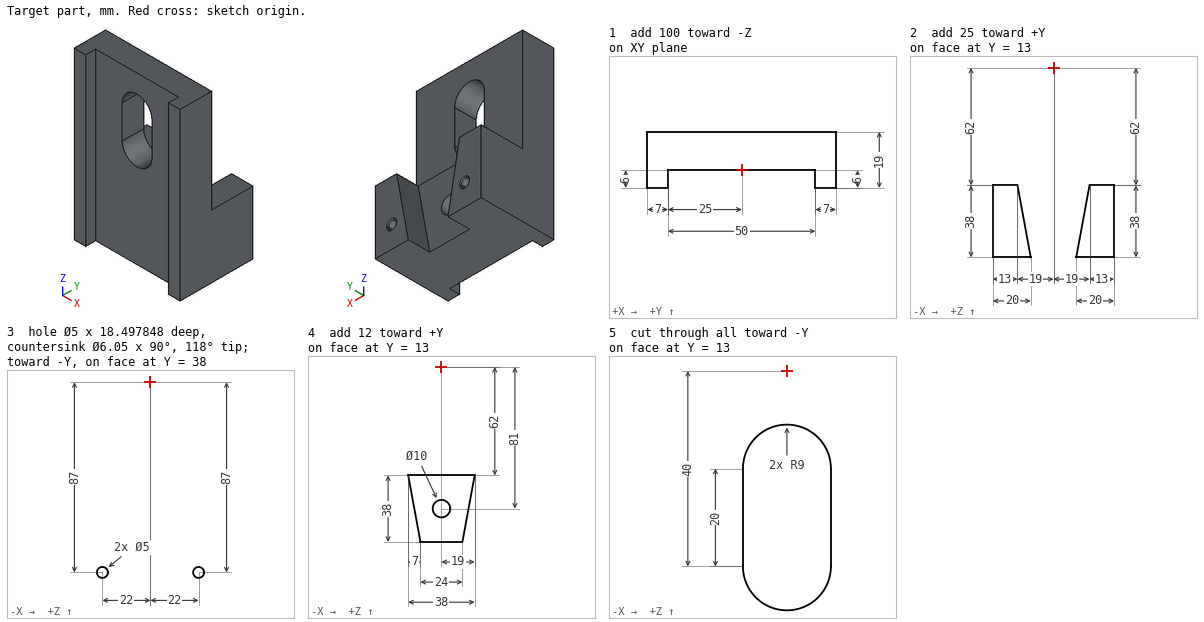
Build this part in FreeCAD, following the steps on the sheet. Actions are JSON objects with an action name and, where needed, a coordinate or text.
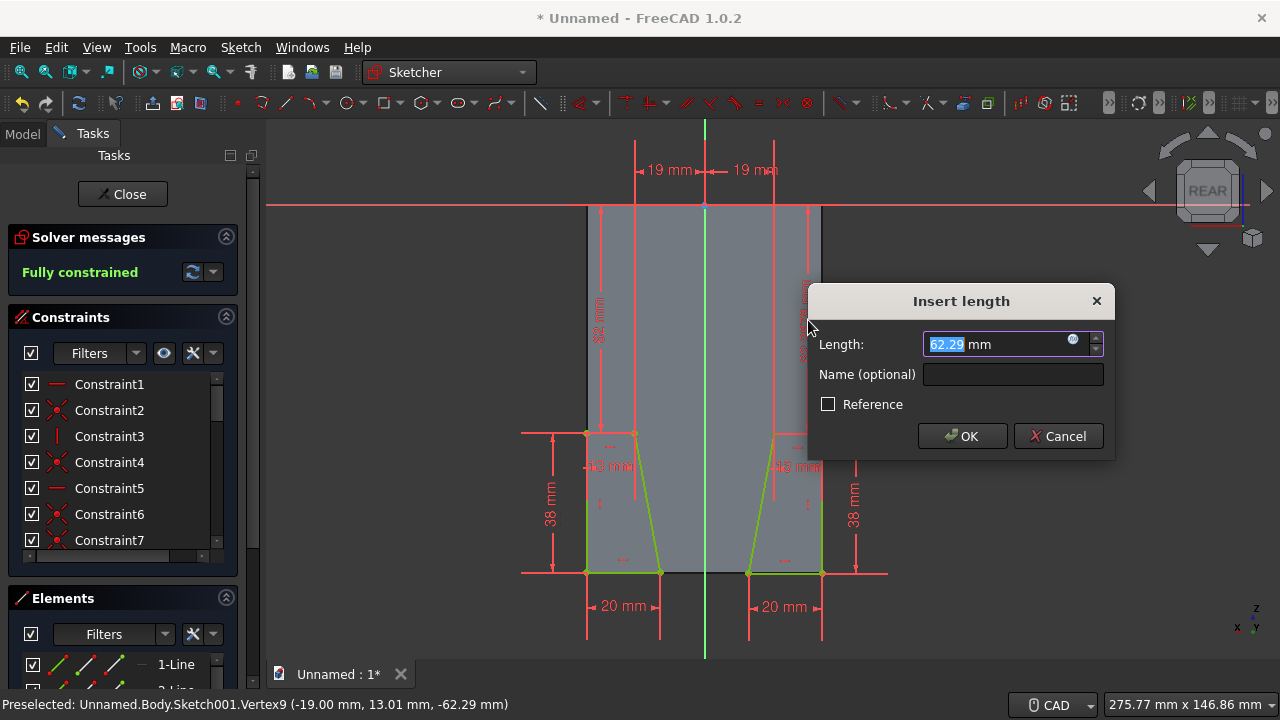
{"action": "type", "text": "62"}
{"action": "key", "text": "Return"}
{"action": "key", "text": "Escape"}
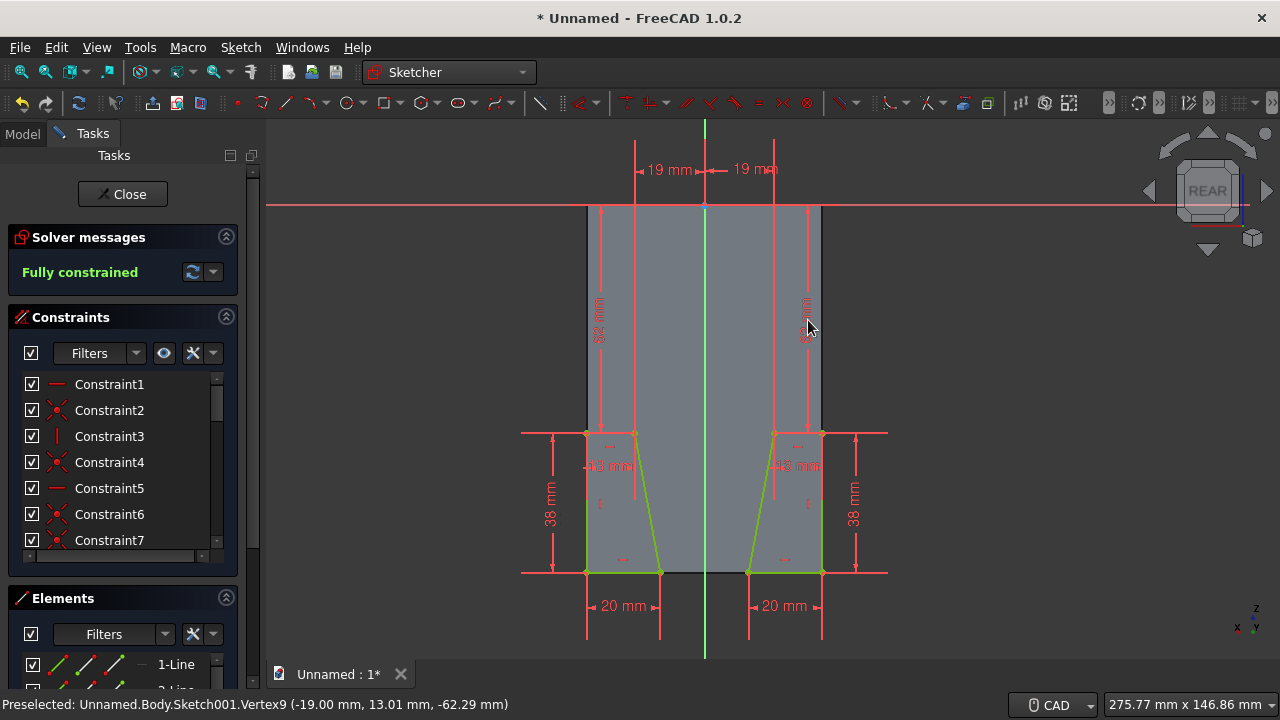
{"action": "left_click", "coordinate": [123, 194]}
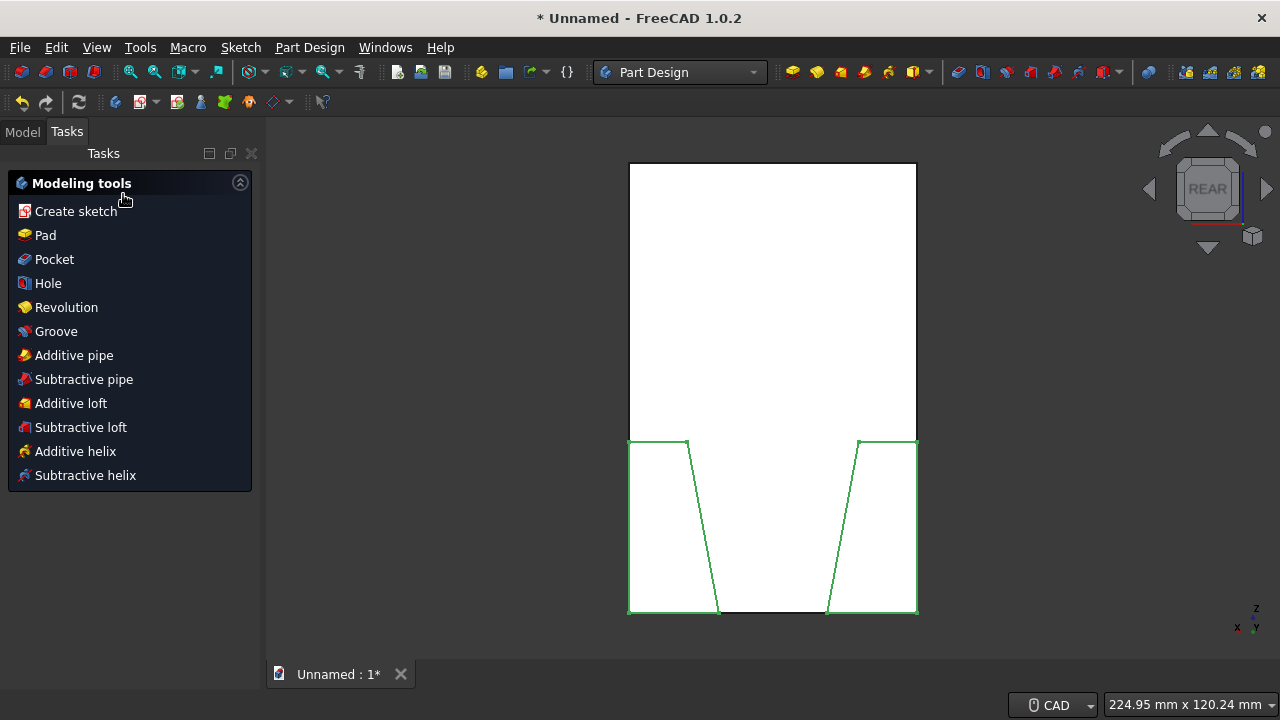
{"action": "left_click", "coordinate": [794, 72]}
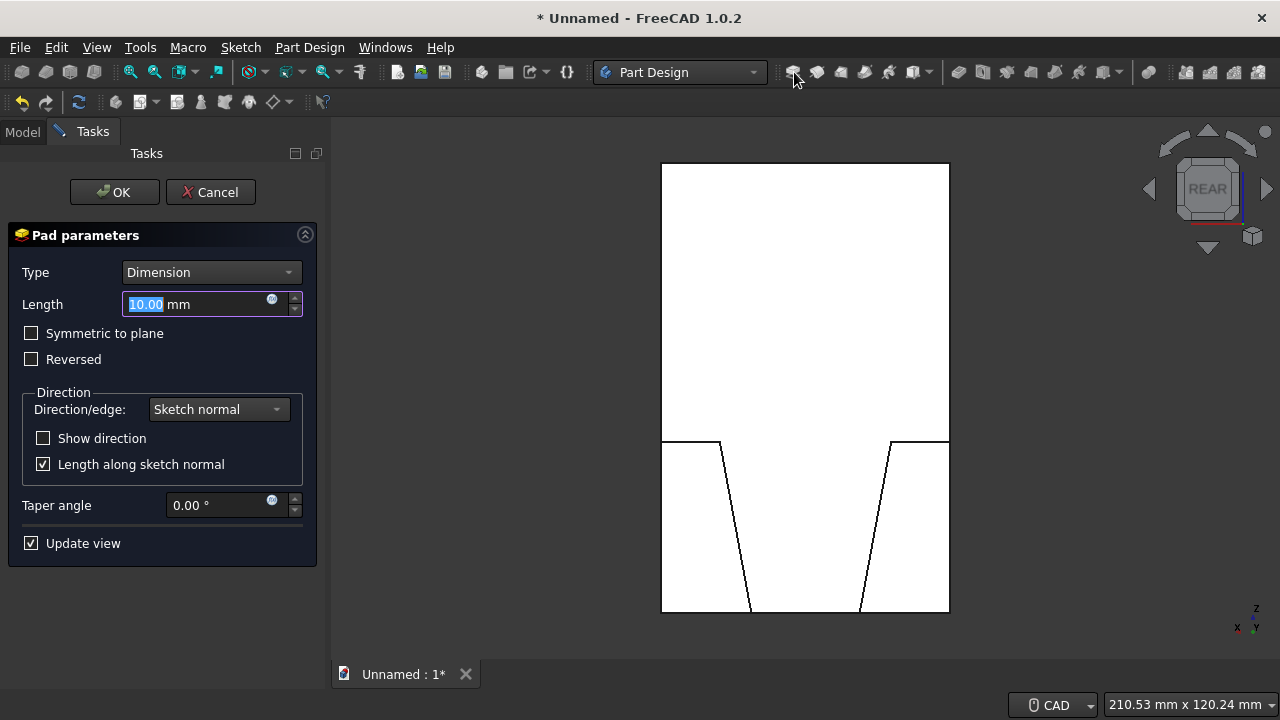
{"action": "type", "text": "25"}
{"action": "key", "text": "Tab"}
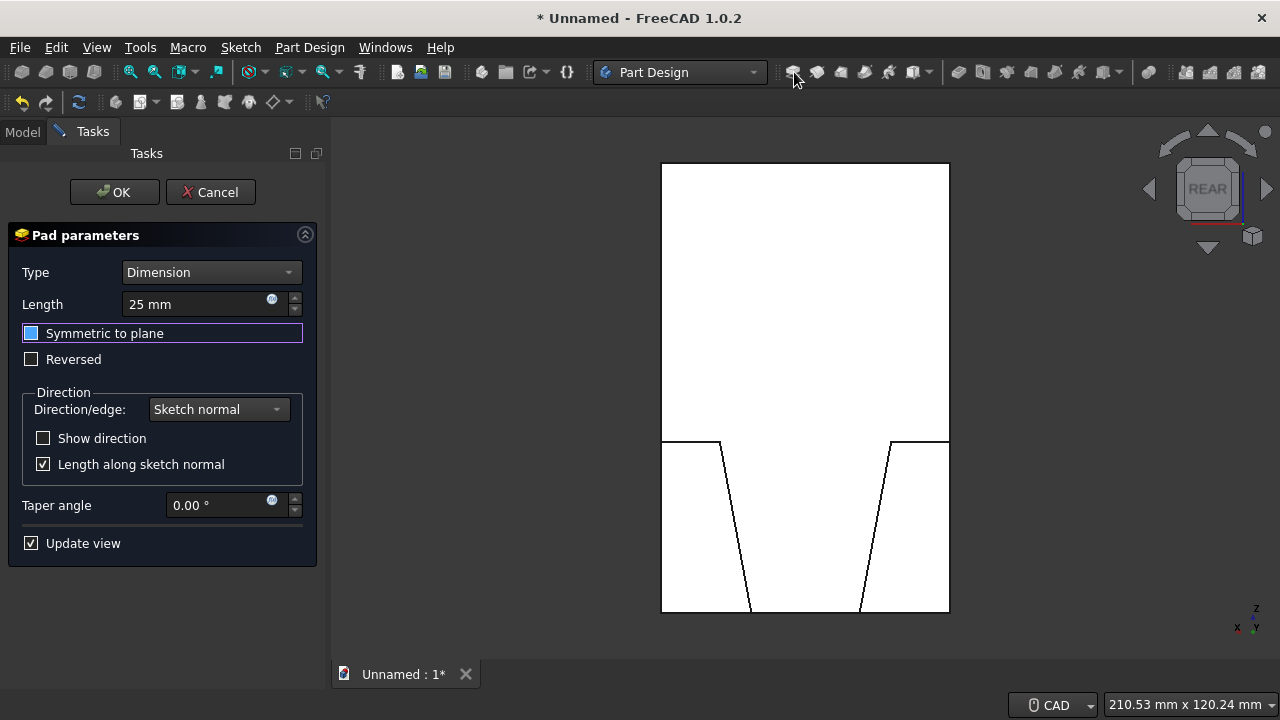
{"action": "left_click", "coordinate": [115, 192]}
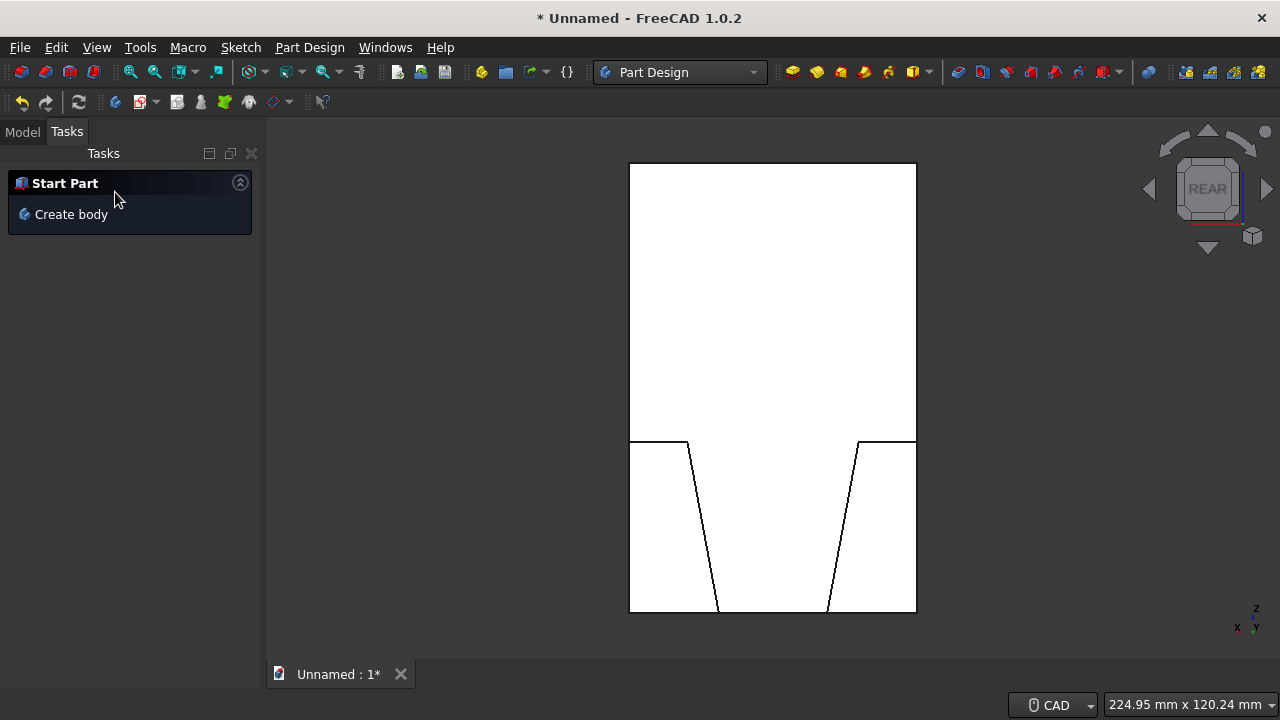
{"action": "left_click", "coordinate": [872, 576]}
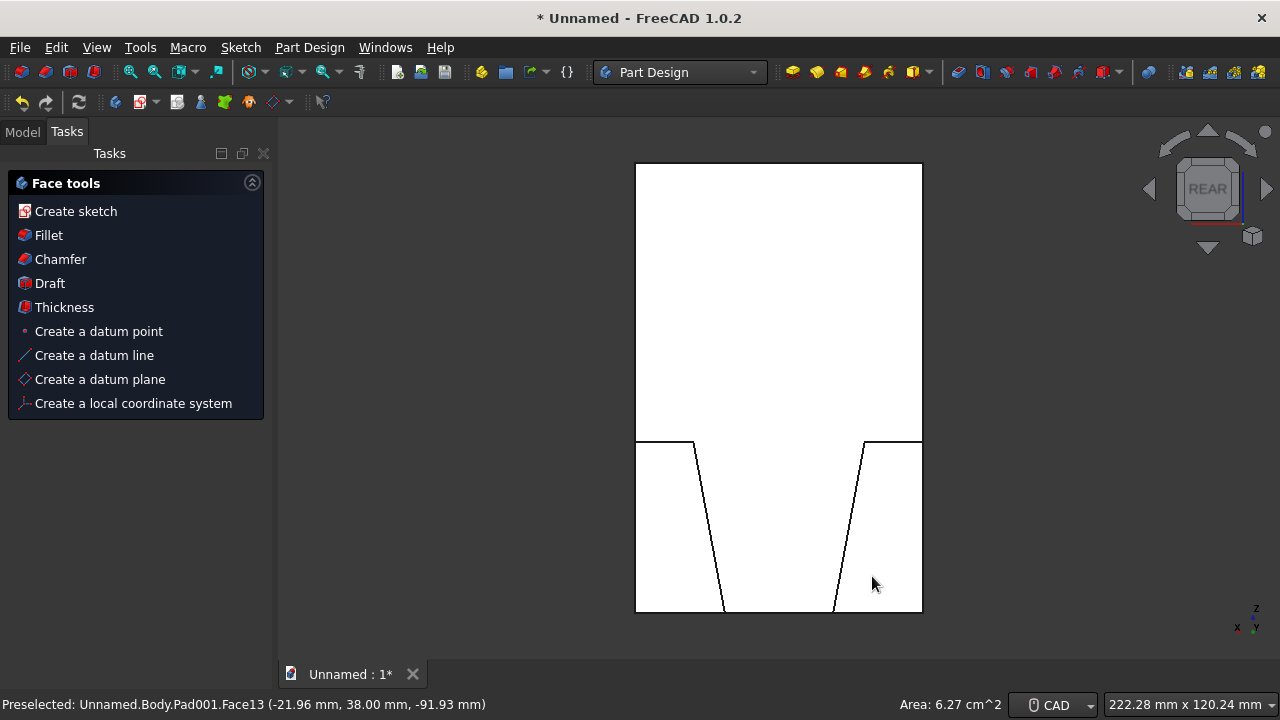
{"action": "left_click", "coordinate": [140, 102]}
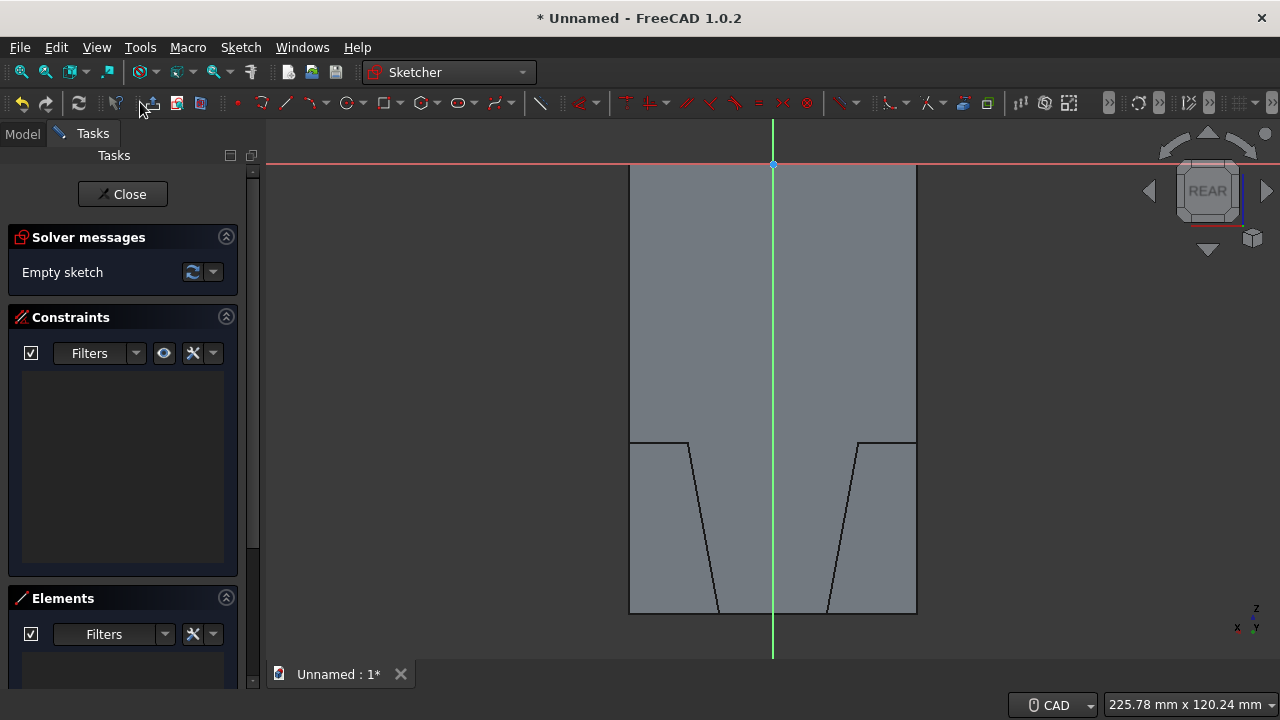
{"action": "scroll", "coordinate": [395, 495], "scroll_direction": "down", "scroll_amount": 1}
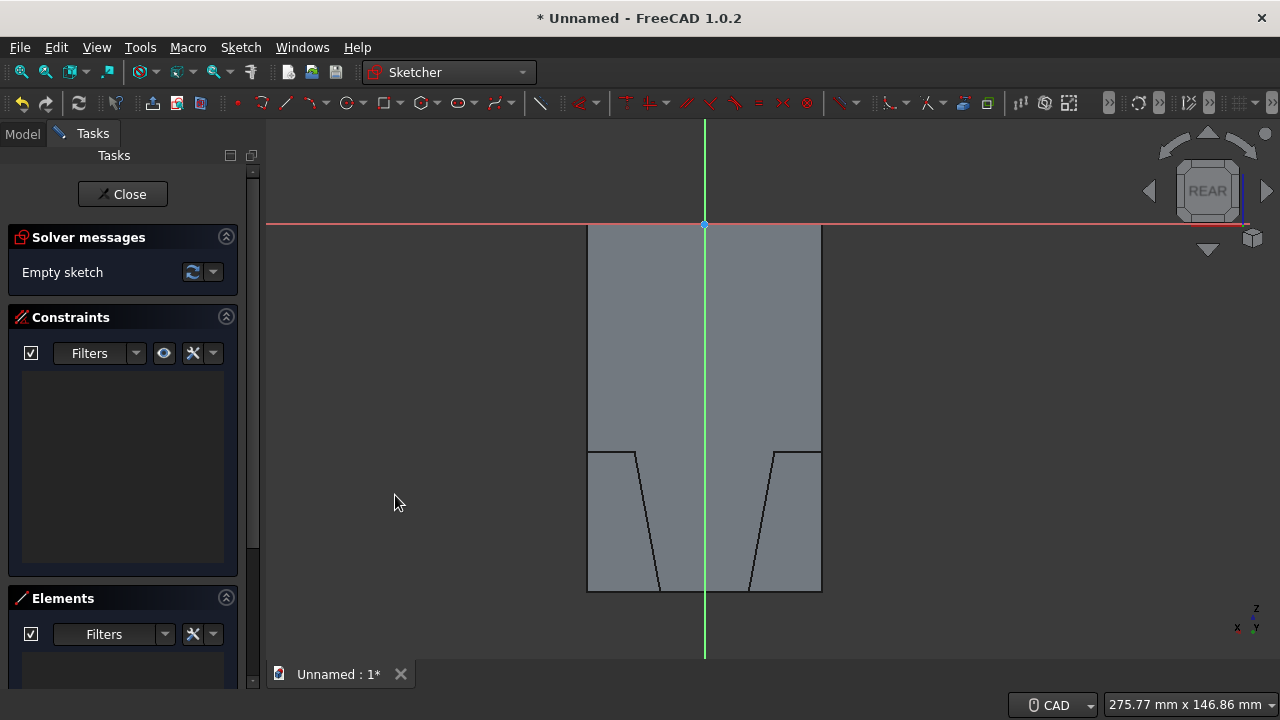
{"action": "key", "text": "g c"}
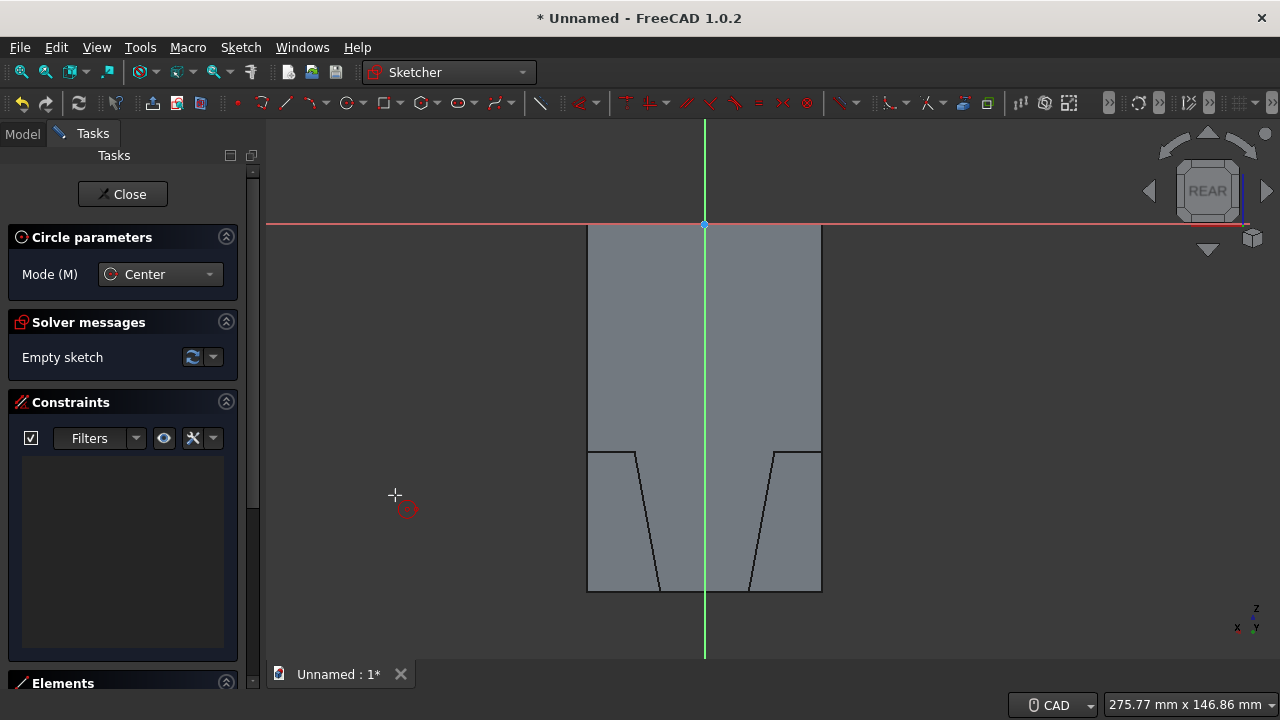
{"action": "scroll", "coordinate": [624, 544], "scroll_direction": "up", "scroll_amount": 5}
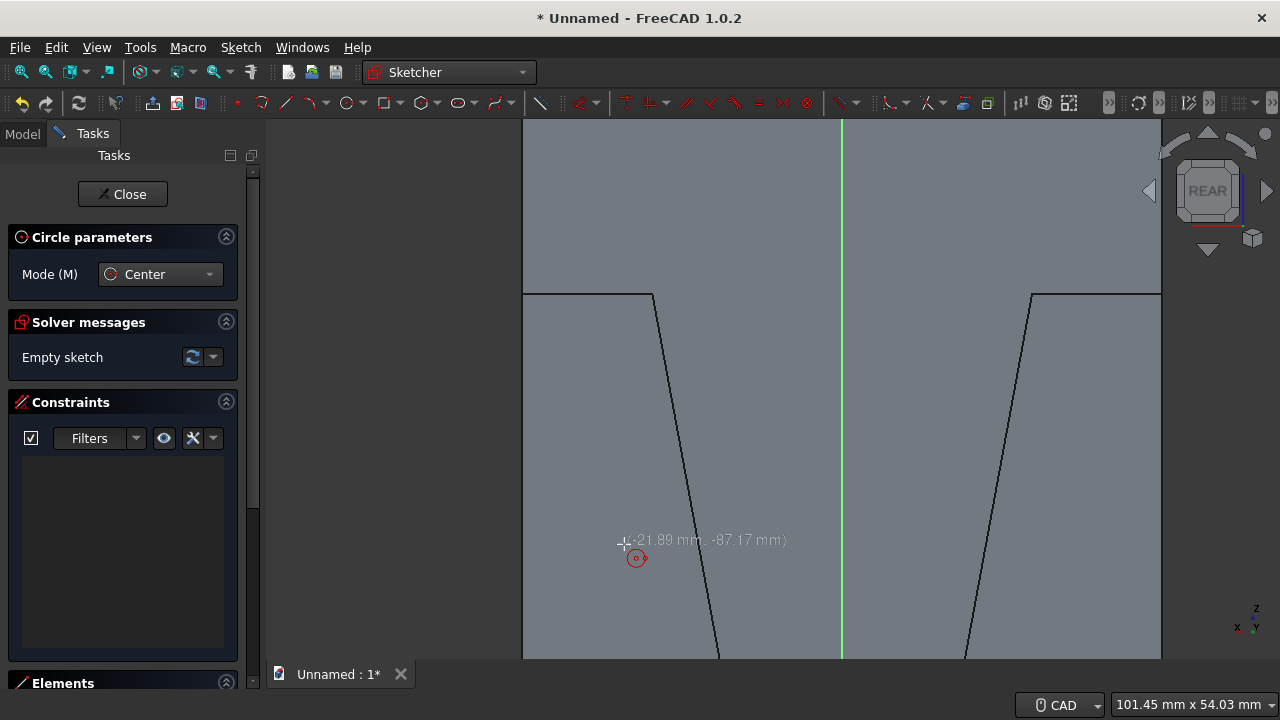
{"action": "left_click", "coordinate": [622, 544]}
{"action": "left_click", "coordinate": [640, 526]}